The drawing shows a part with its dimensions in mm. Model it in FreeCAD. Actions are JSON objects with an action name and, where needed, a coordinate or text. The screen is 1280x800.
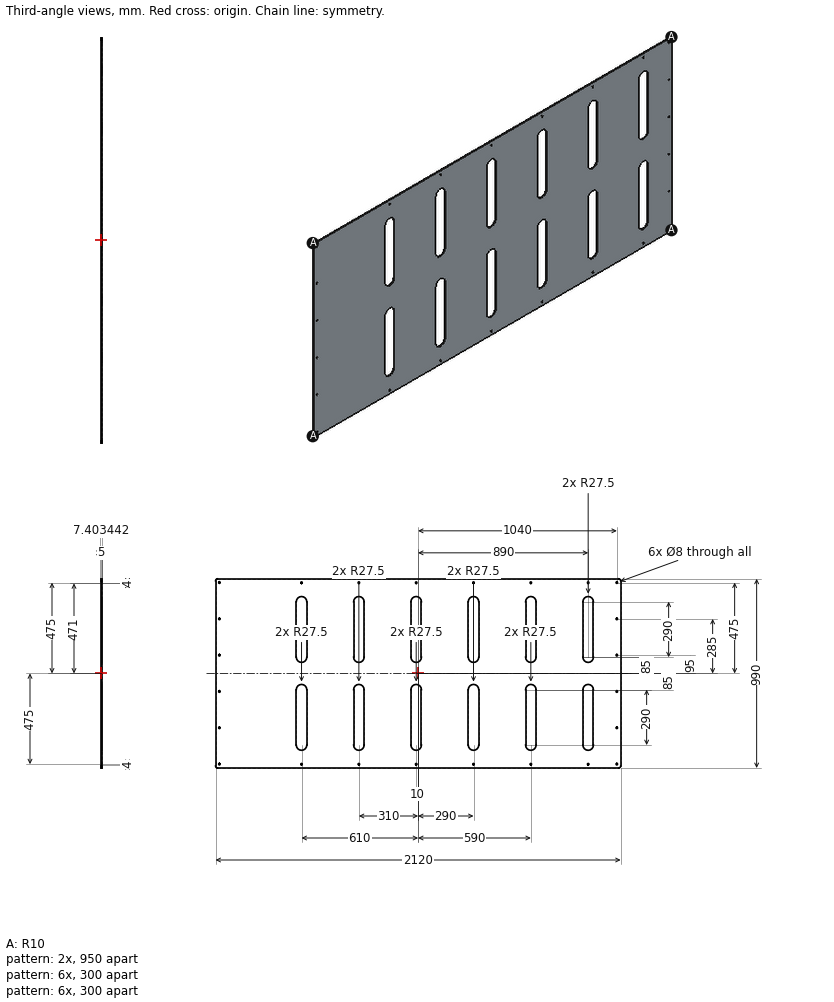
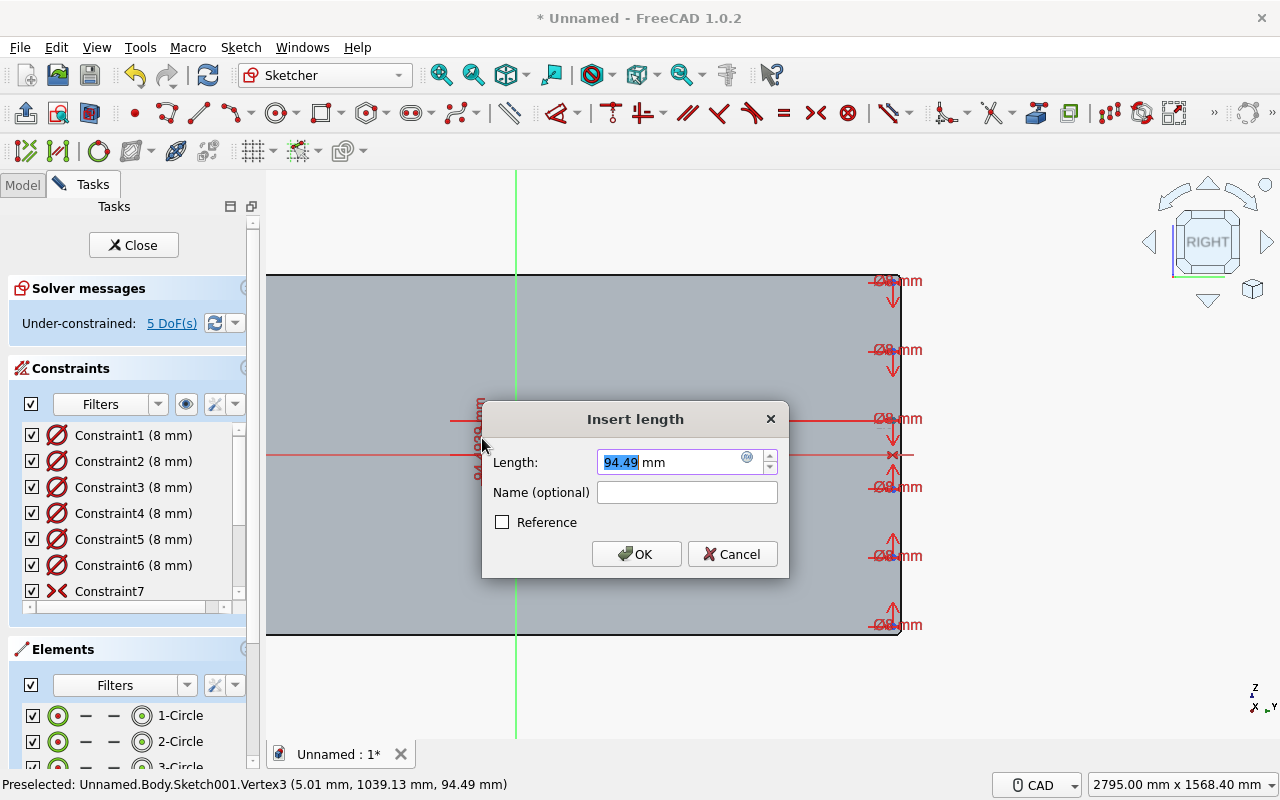
{"action": "type", "text": "95"}
{"action": "key", "text": "Return"}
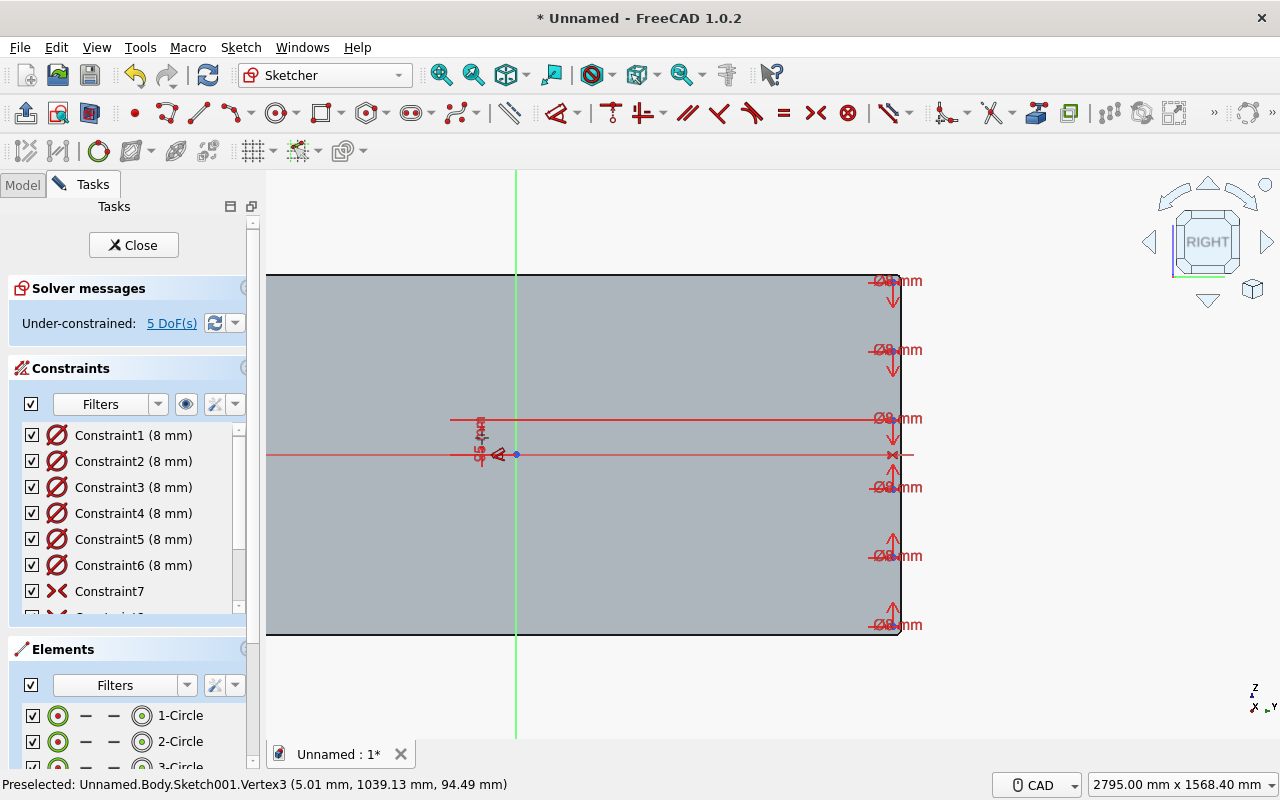
{"action": "left_click", "coordinate": [893, 283]}
{"action": "left_click", "coordinate": [482, 369]}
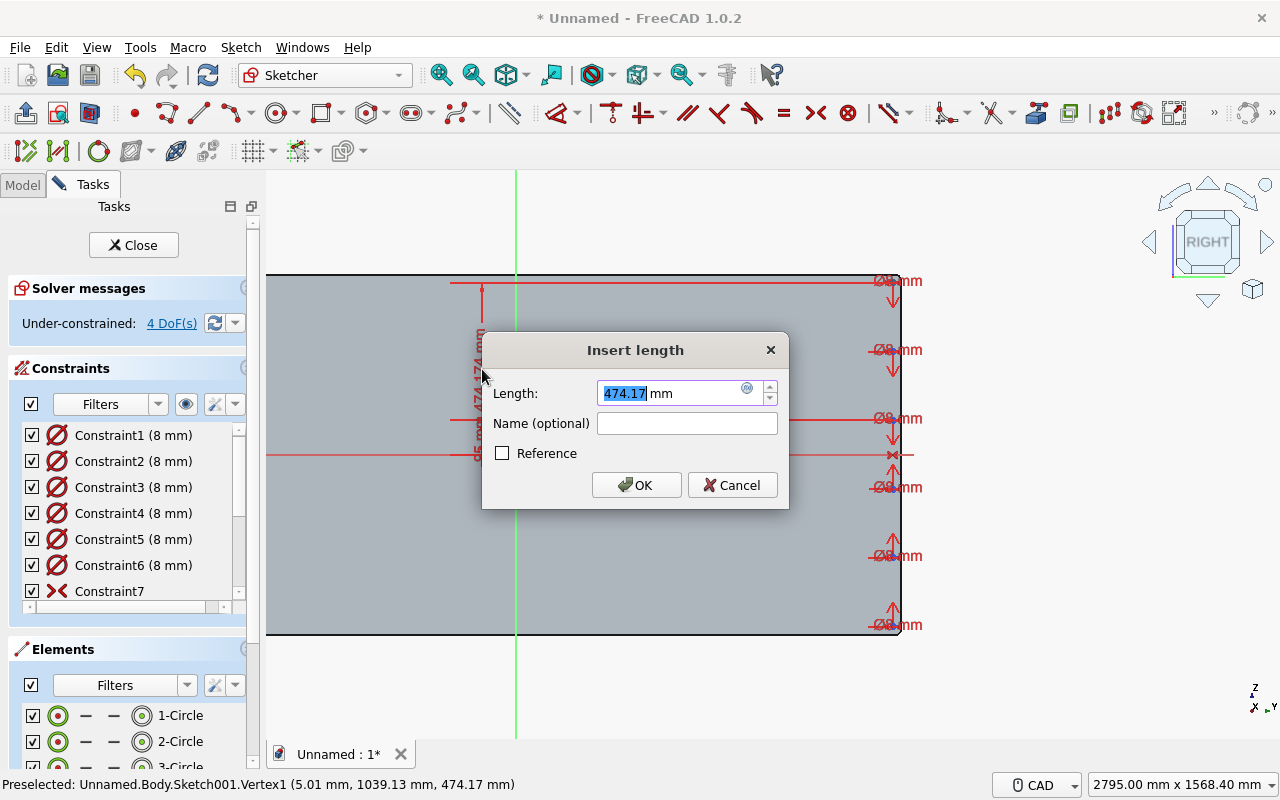
{"action": "type", "text": "475"}
{"action": "key", "text": "Return"}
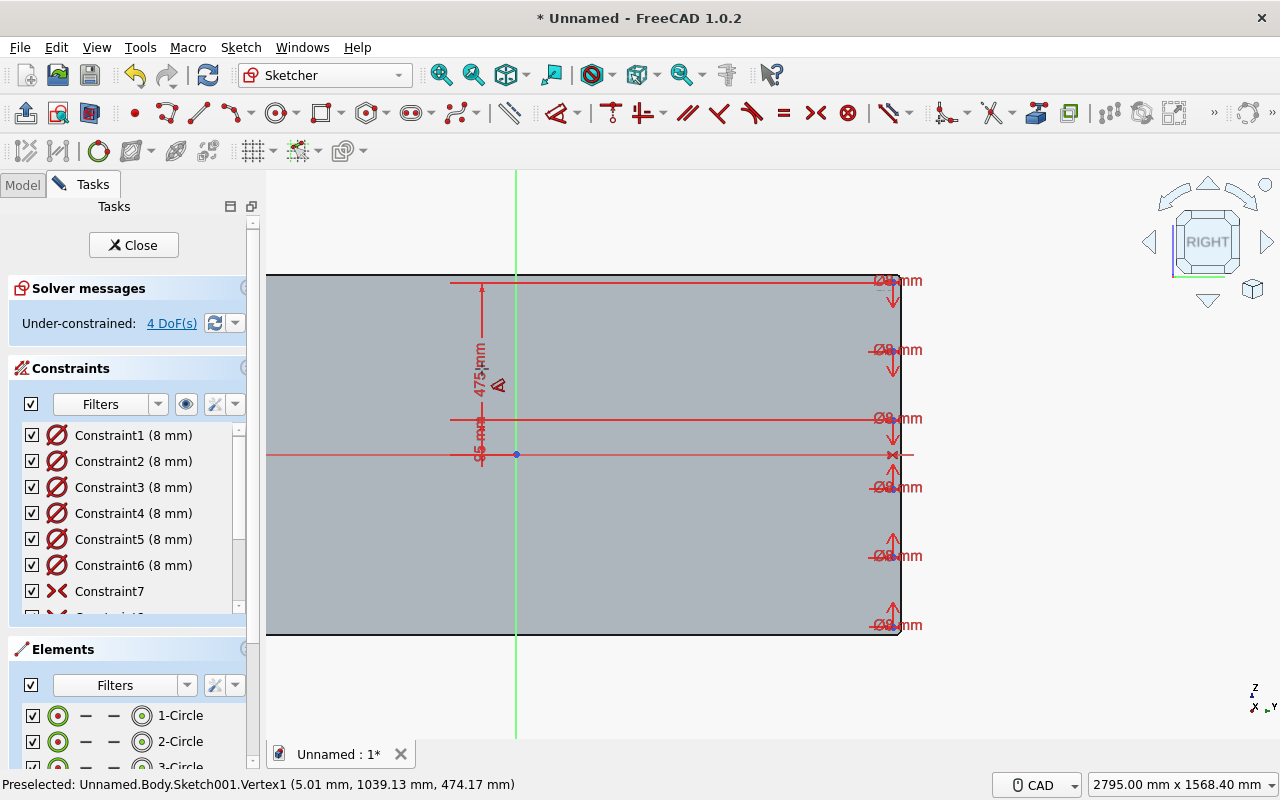
{"action": "left_click", "coordinate": [893, 352]}
{"action": "left_click", "coordinate": [482, 403]}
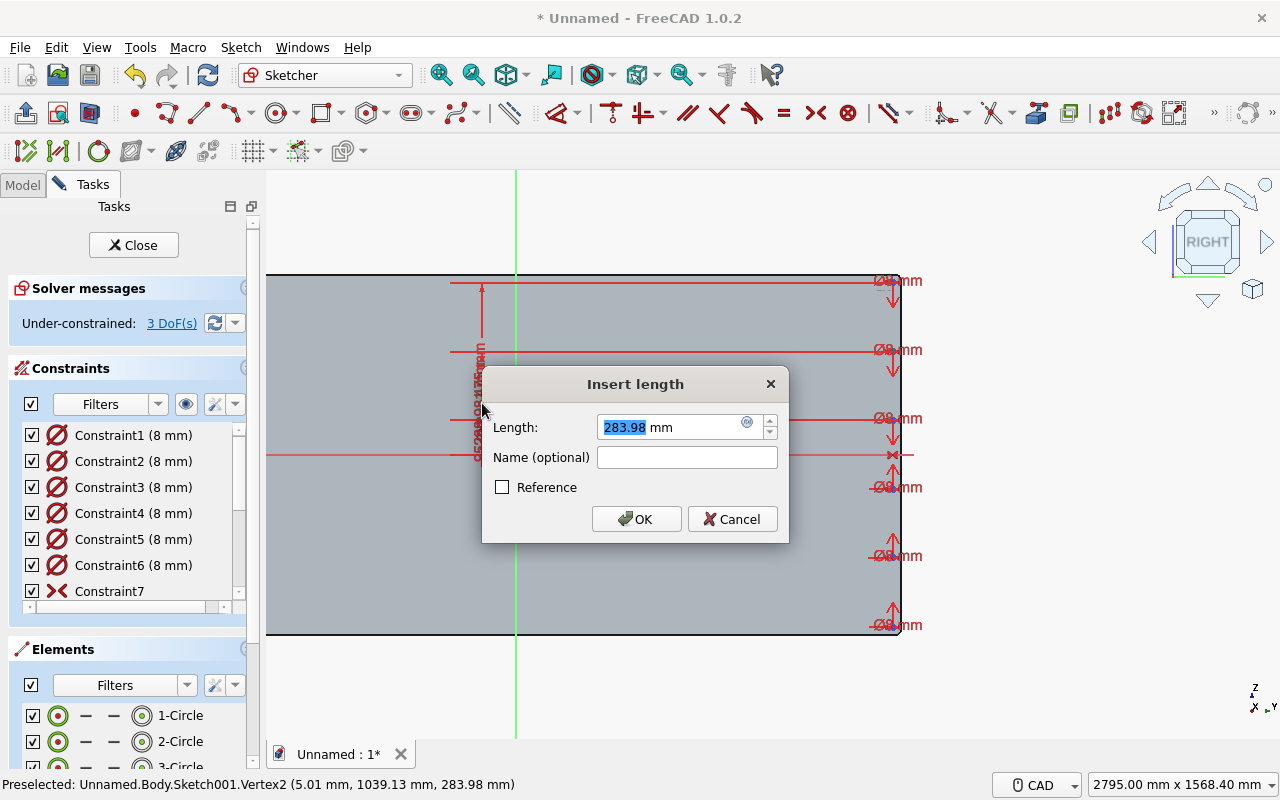
{"action": "type", "text": "285"}
{"action": "key", "text": "Return"}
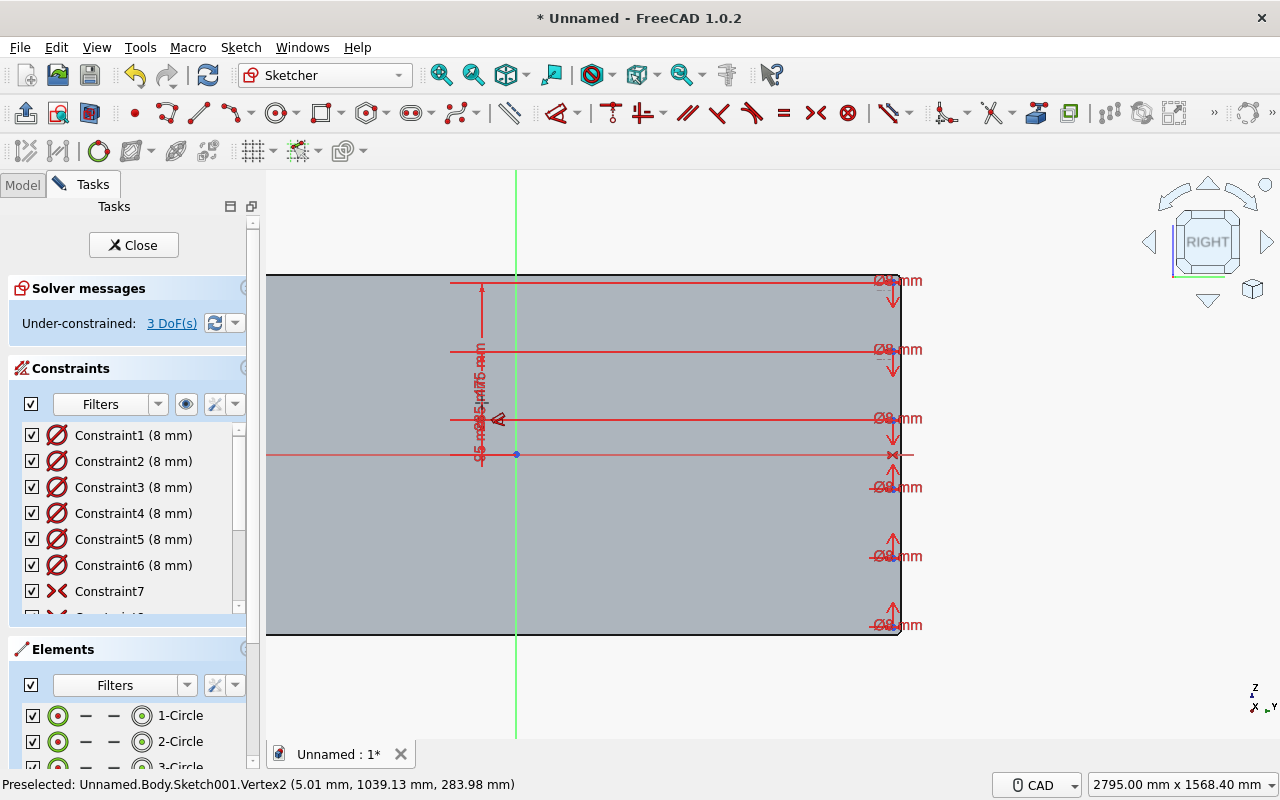
{"action": "left_click", "coordinate": [893, 283]}
{"action": "left_click", "coordinate": [705, 249]}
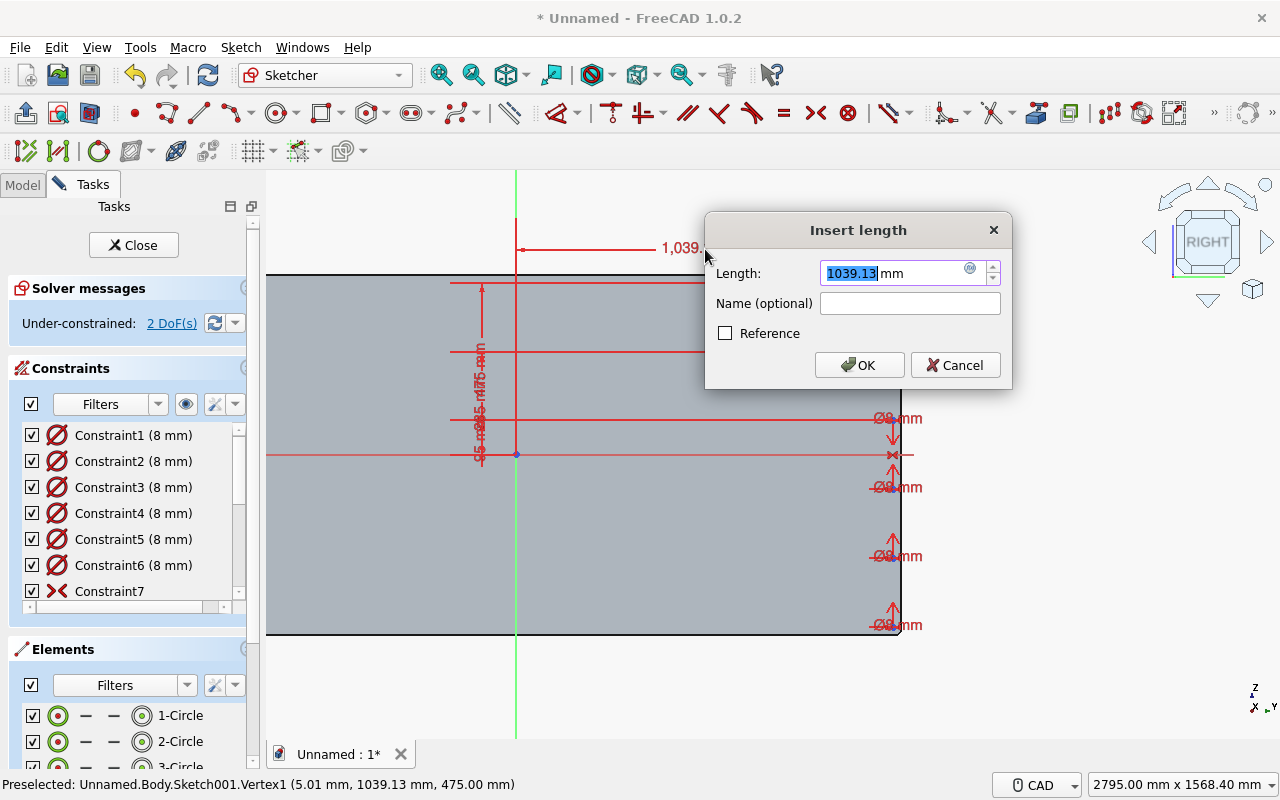
{"action": "type", "text": "1040"}
{"action": "key", "text": "Return"}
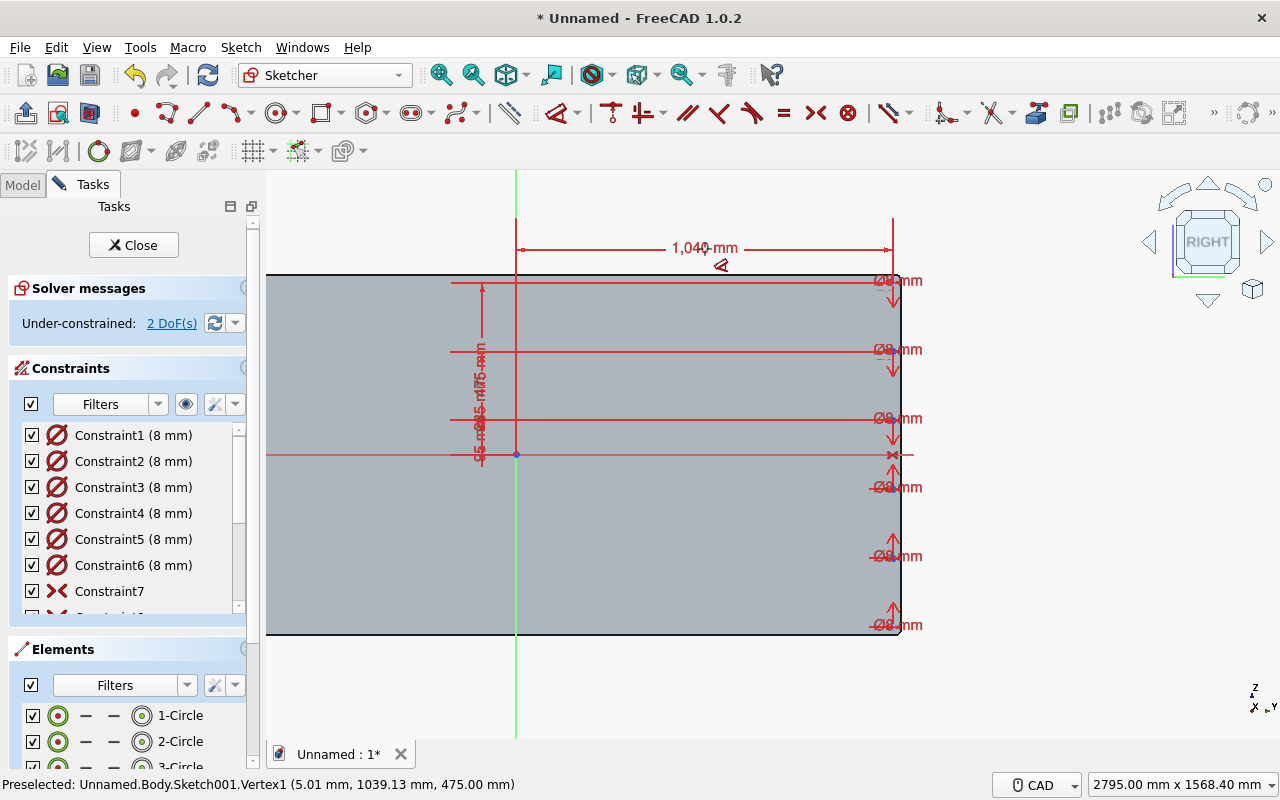
{"action": "left_click", "coordinate": [893, 352]}
{"action": "left_click", "coordinate": [705, 318]}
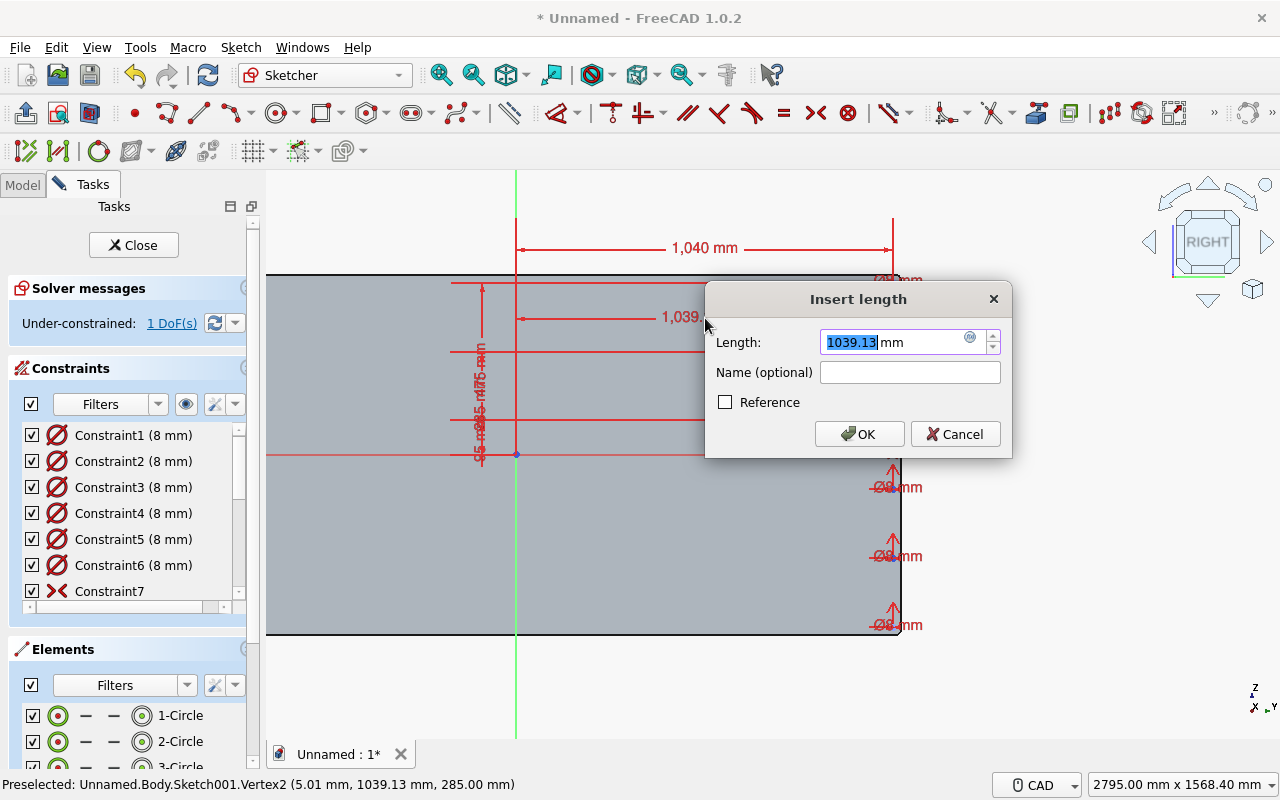
{"action": "type", "text": "1040"}
{"action": "key", "text": "Return"}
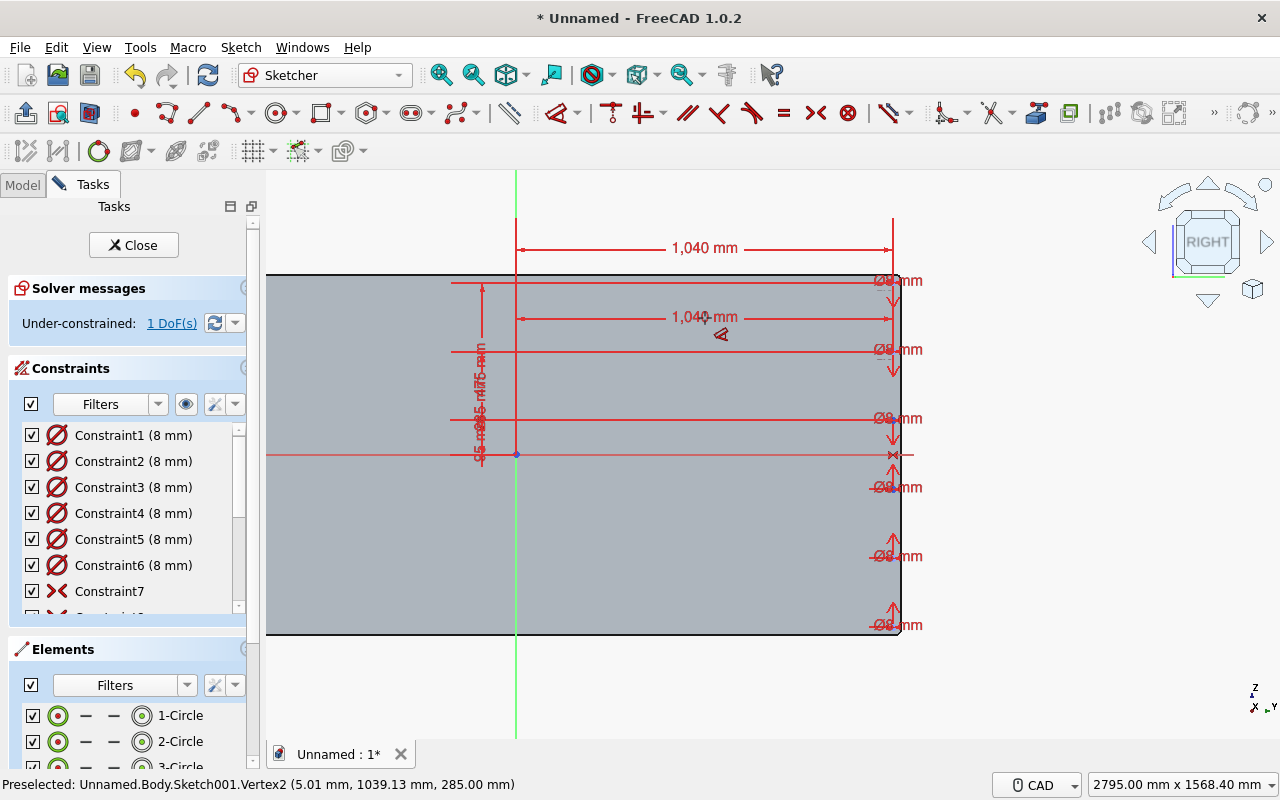
{"action": "left_click", "coordinate": [893, 420]}
{"action": "left_click", "coordinate": [705, 386]}